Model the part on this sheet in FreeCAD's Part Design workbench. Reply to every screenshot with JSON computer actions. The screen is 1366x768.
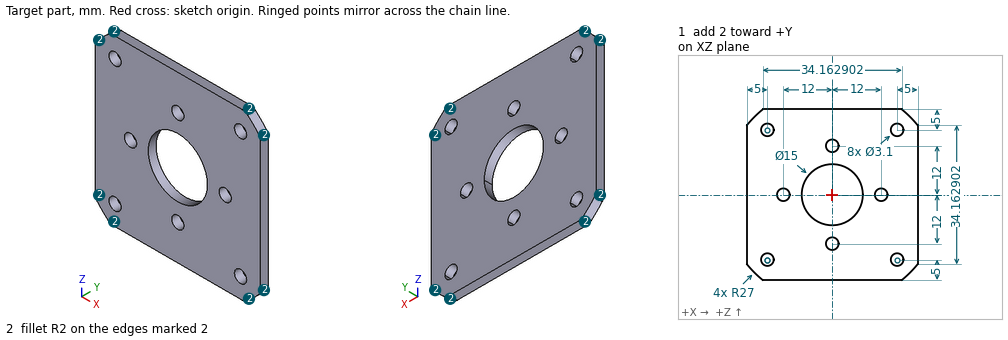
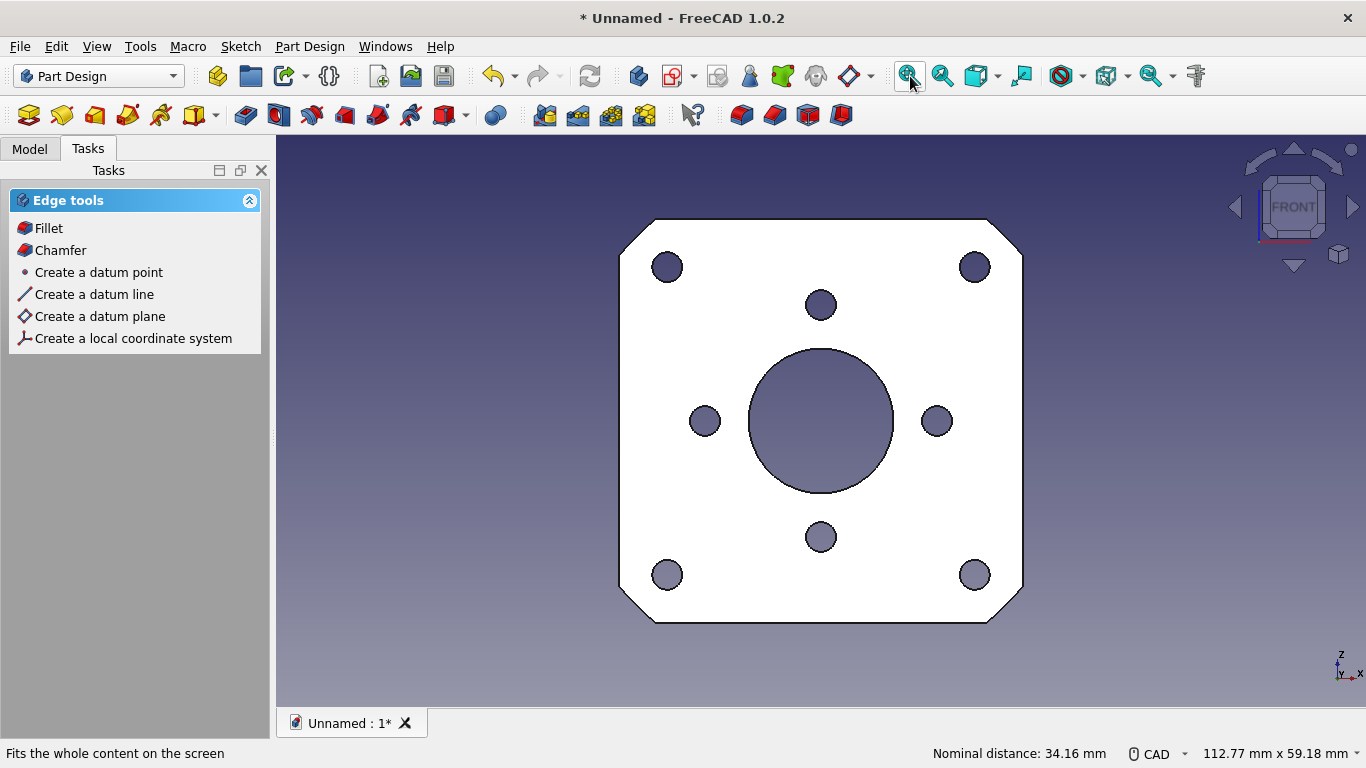
{"action": "scroll", "coordinate": [619, 255], "scroll_direction": "up", "scroll_amount": 4}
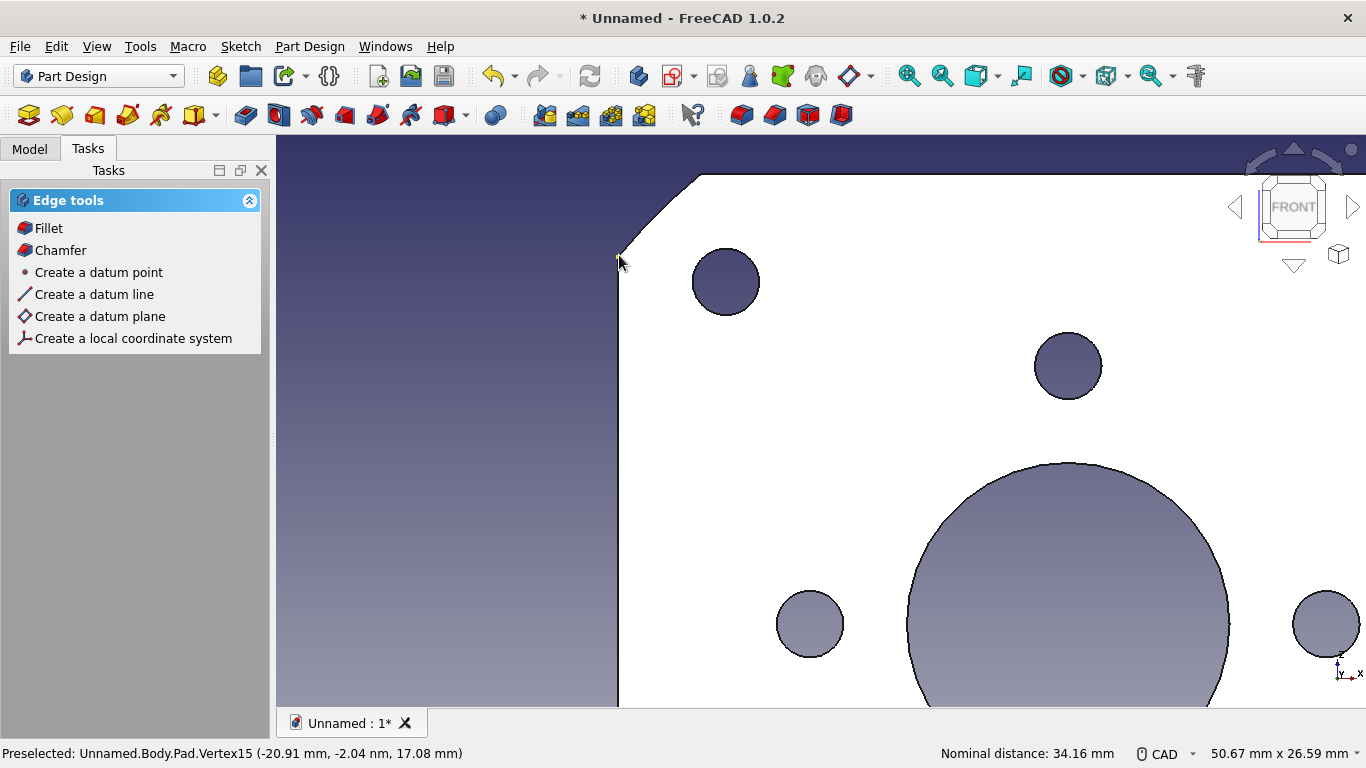
{"action": "left_click", "coordinate": [910, 76]}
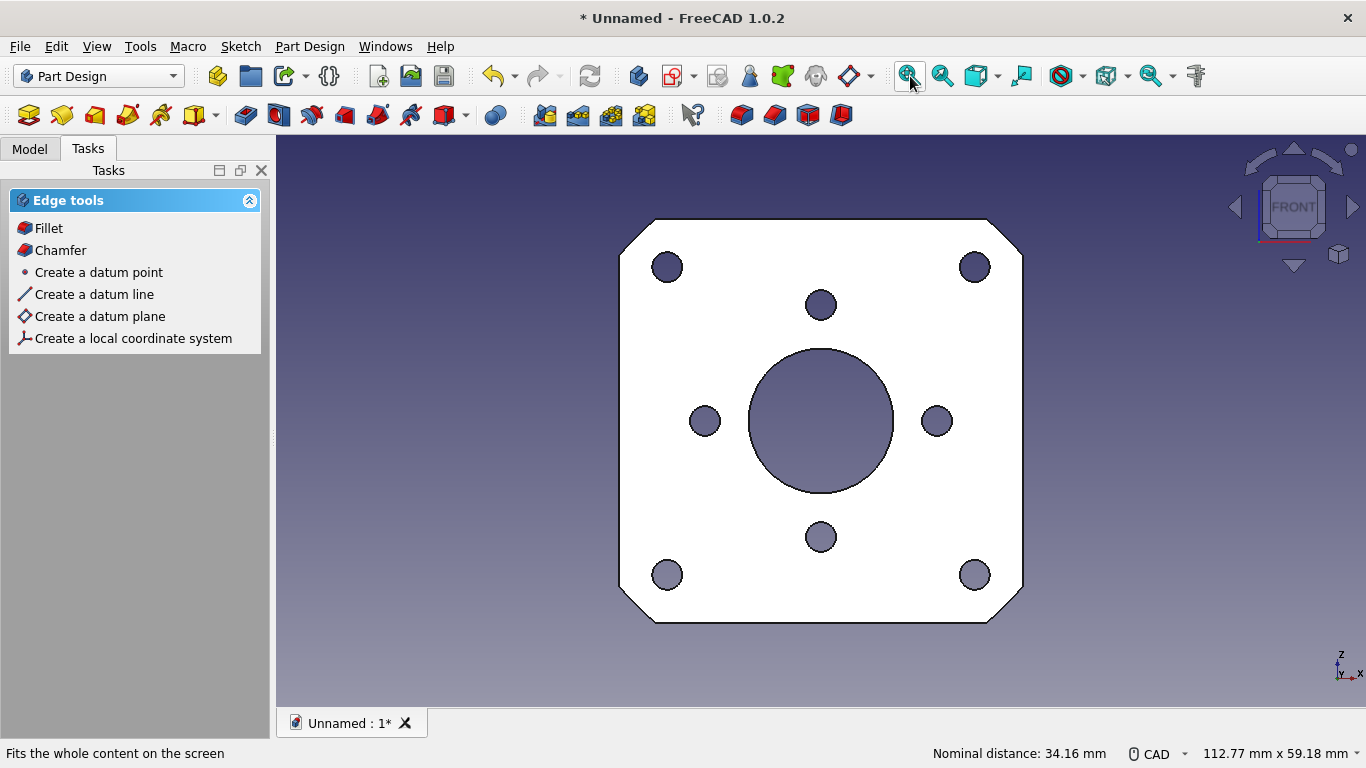
{"action": "key", "text": "3"}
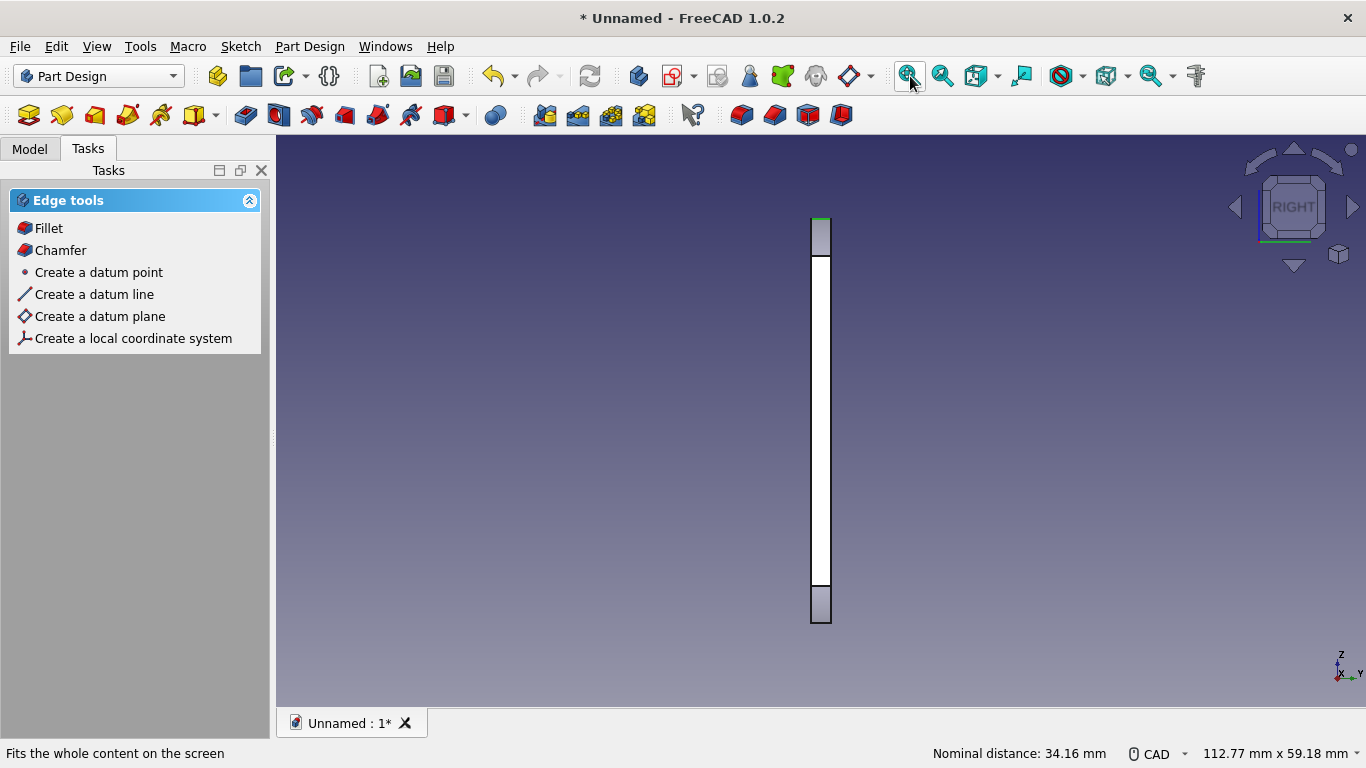
{"action": "left_click", "coordinate": [821, 585], "text": "ctrl"}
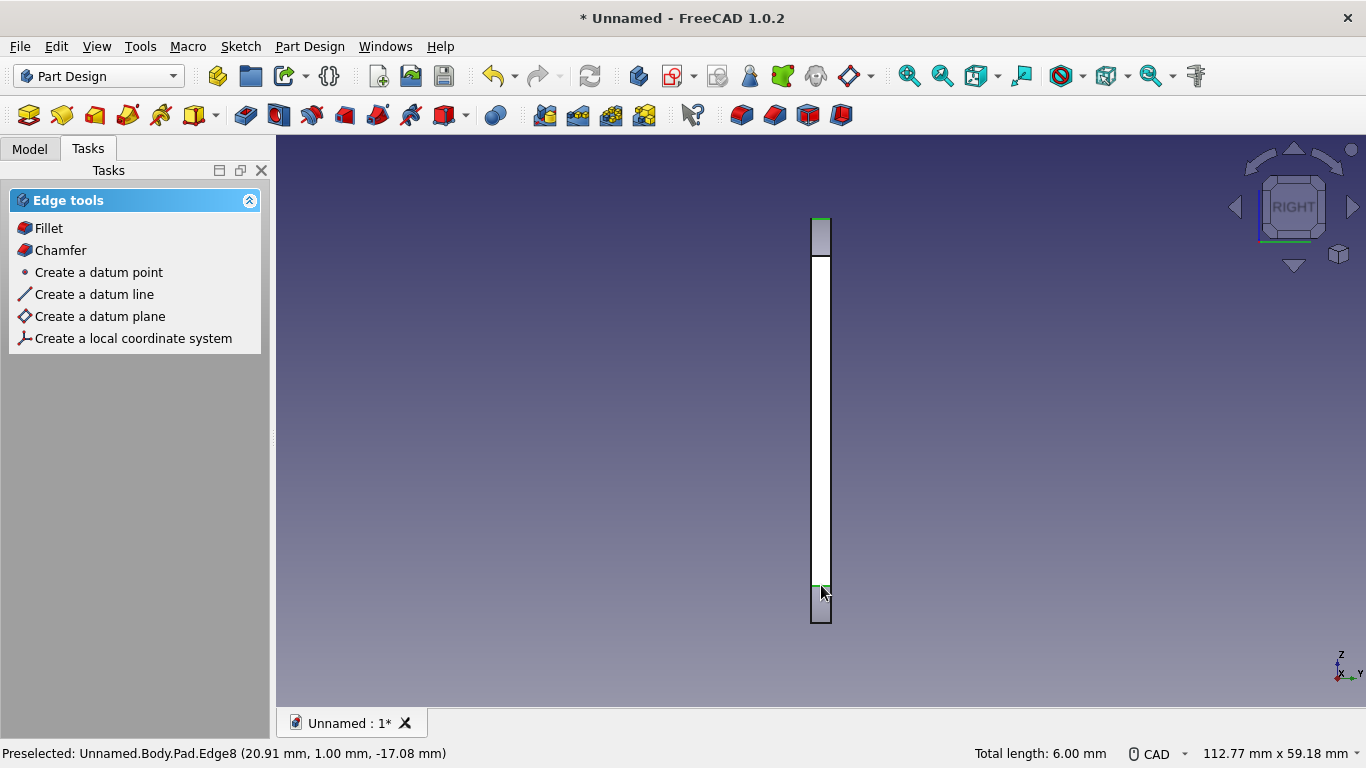
{"action": "left_click", "coordinate": [821, 255], "text": "ctrl"}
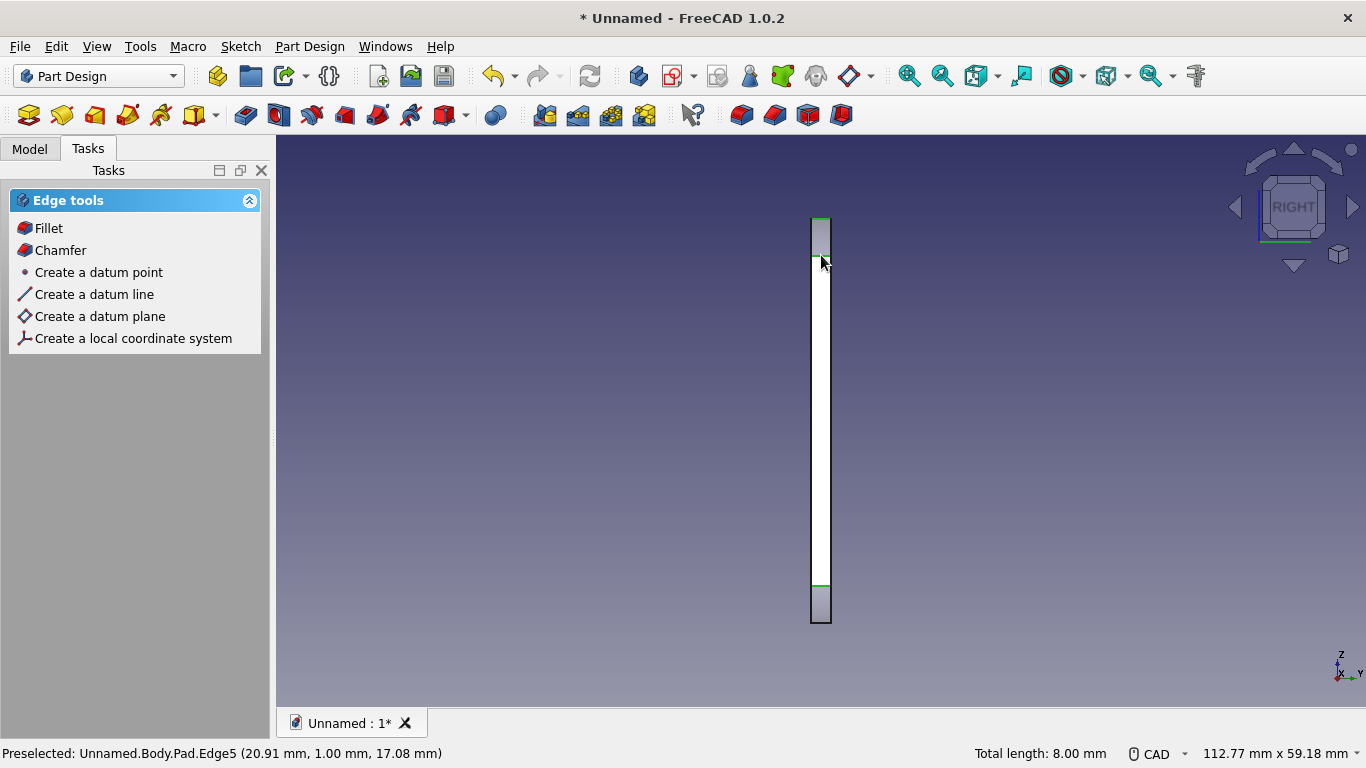
{"action": "scroll", "coordinate": [821, 255], "scroll_direction": "up", "scroll_amount": 4}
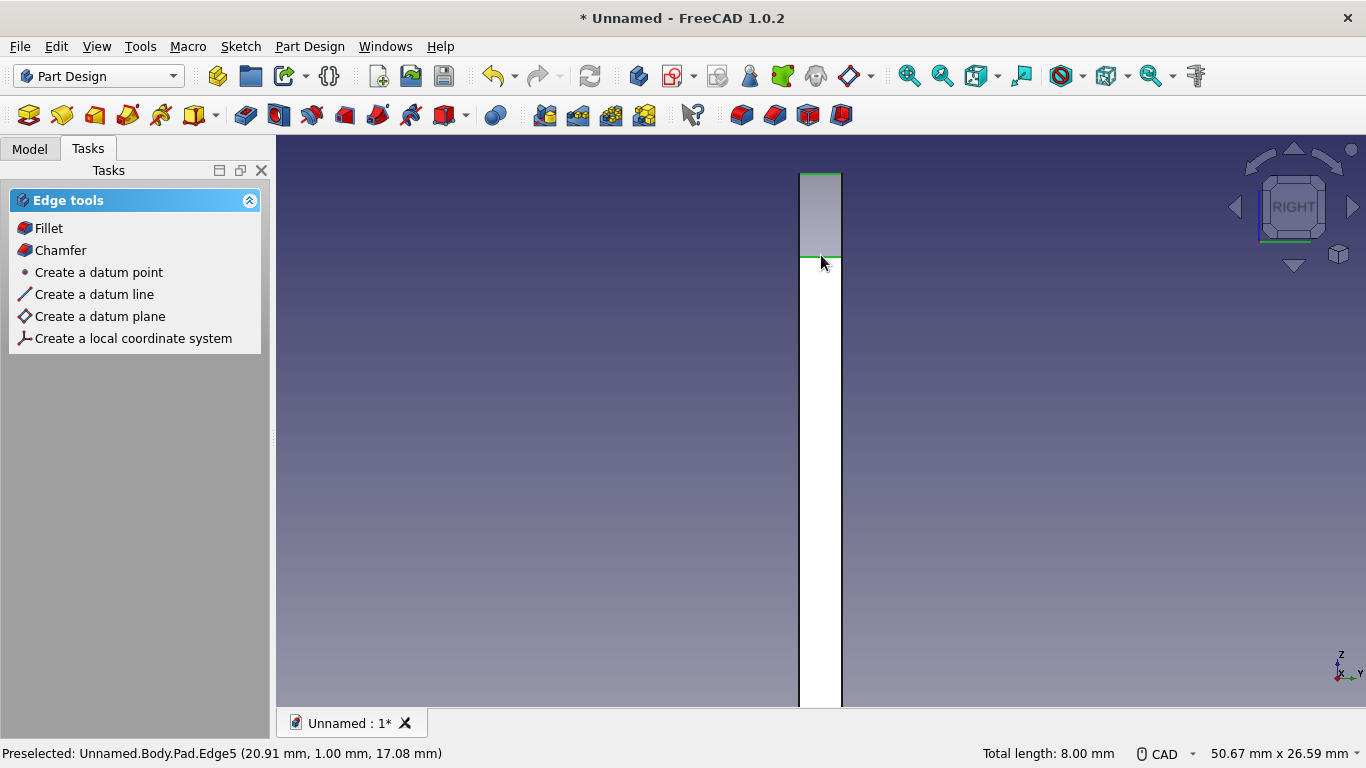
{"action": "left_click", "coordinate": [910, 76]}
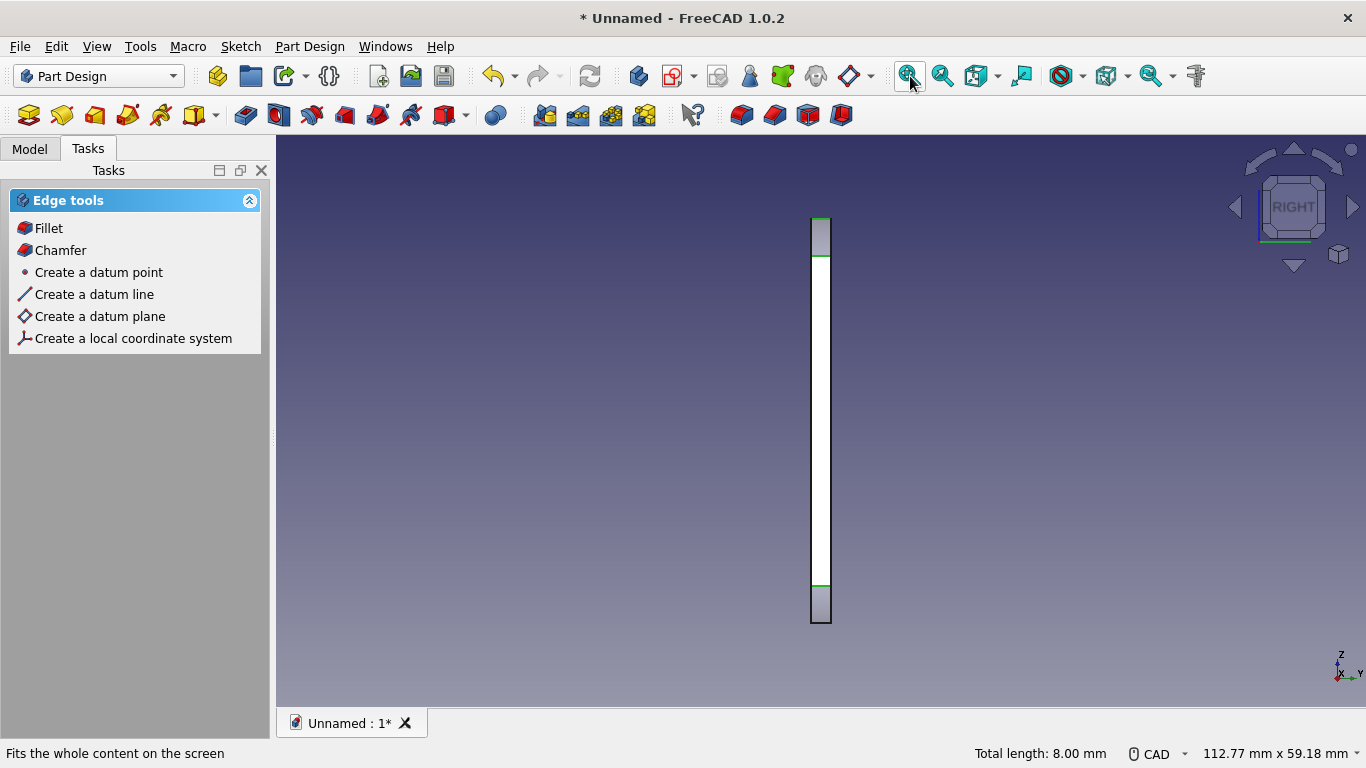
{"action": "key", "text": "5"}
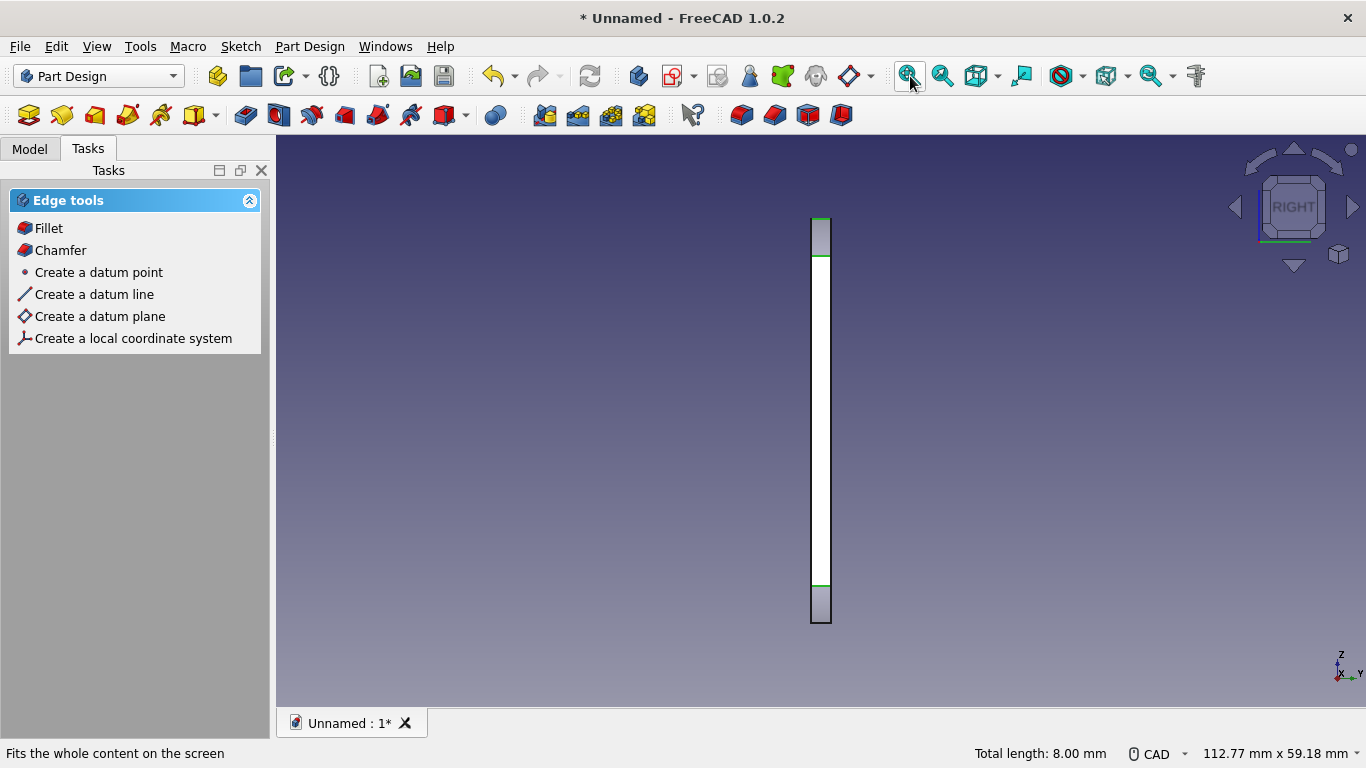
{"action": "left_click", "coordinate": [910, 76]}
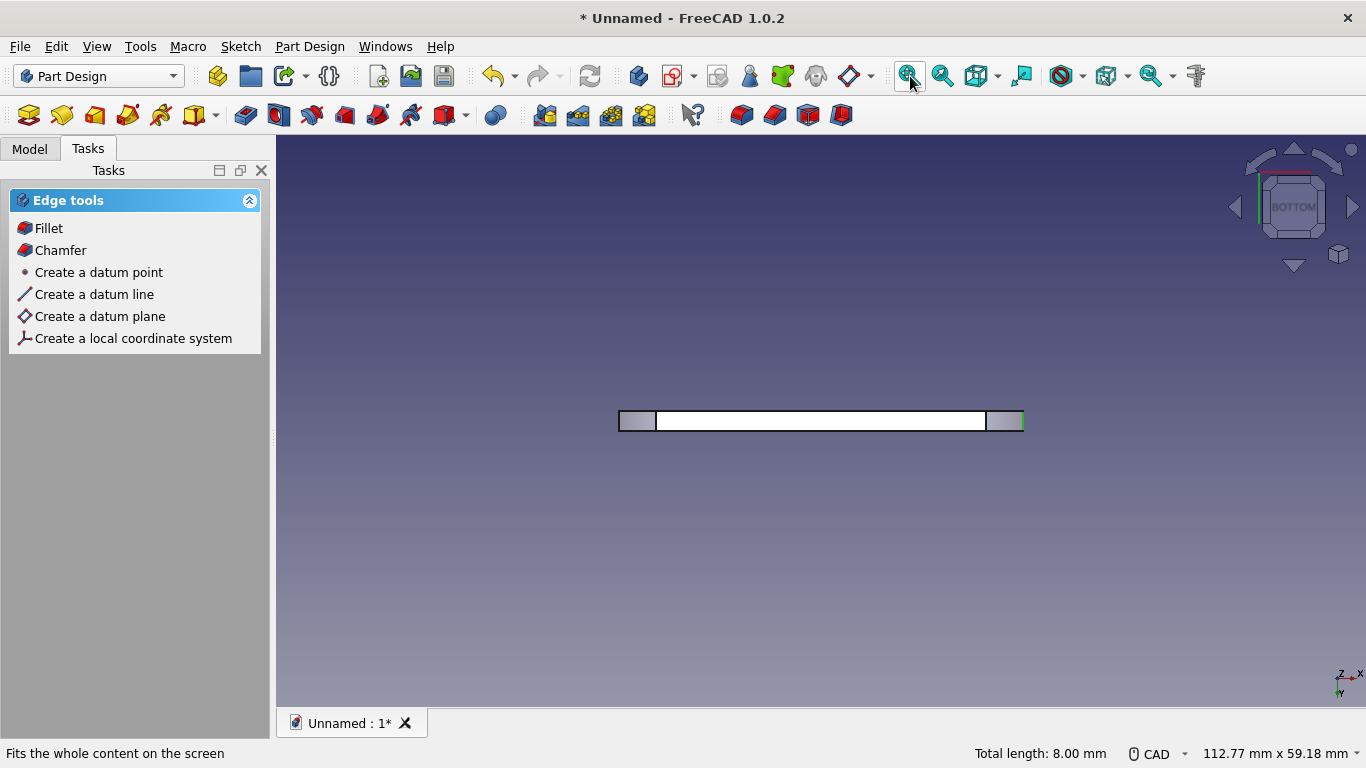
{"action": "left_click", "coordinate": [656, 420], "text": "ctrl"}